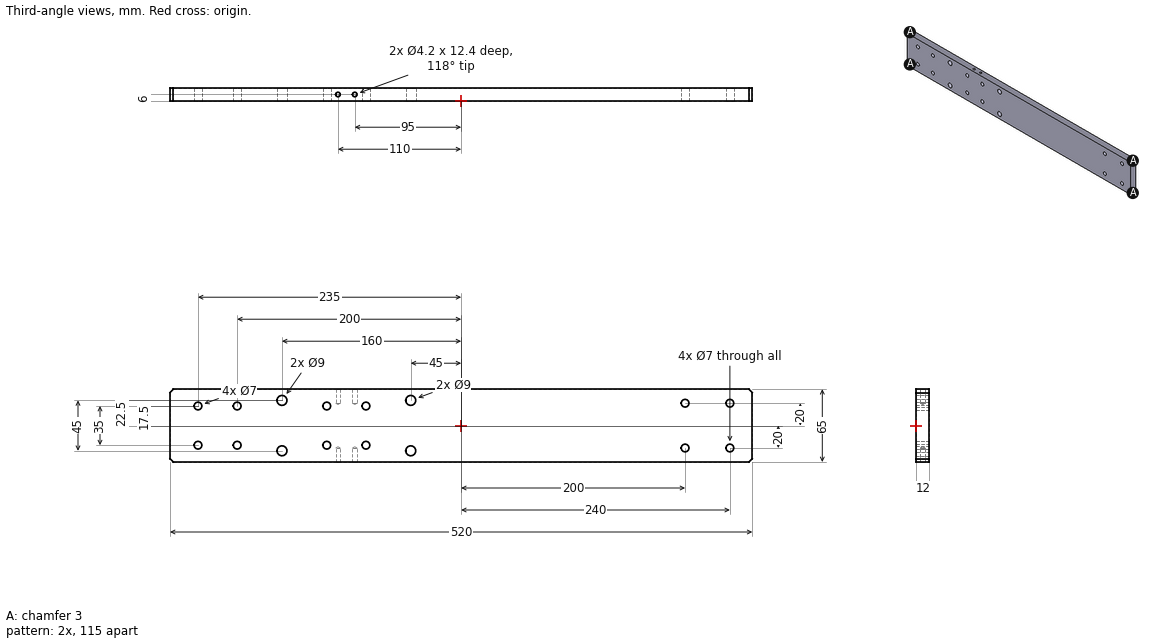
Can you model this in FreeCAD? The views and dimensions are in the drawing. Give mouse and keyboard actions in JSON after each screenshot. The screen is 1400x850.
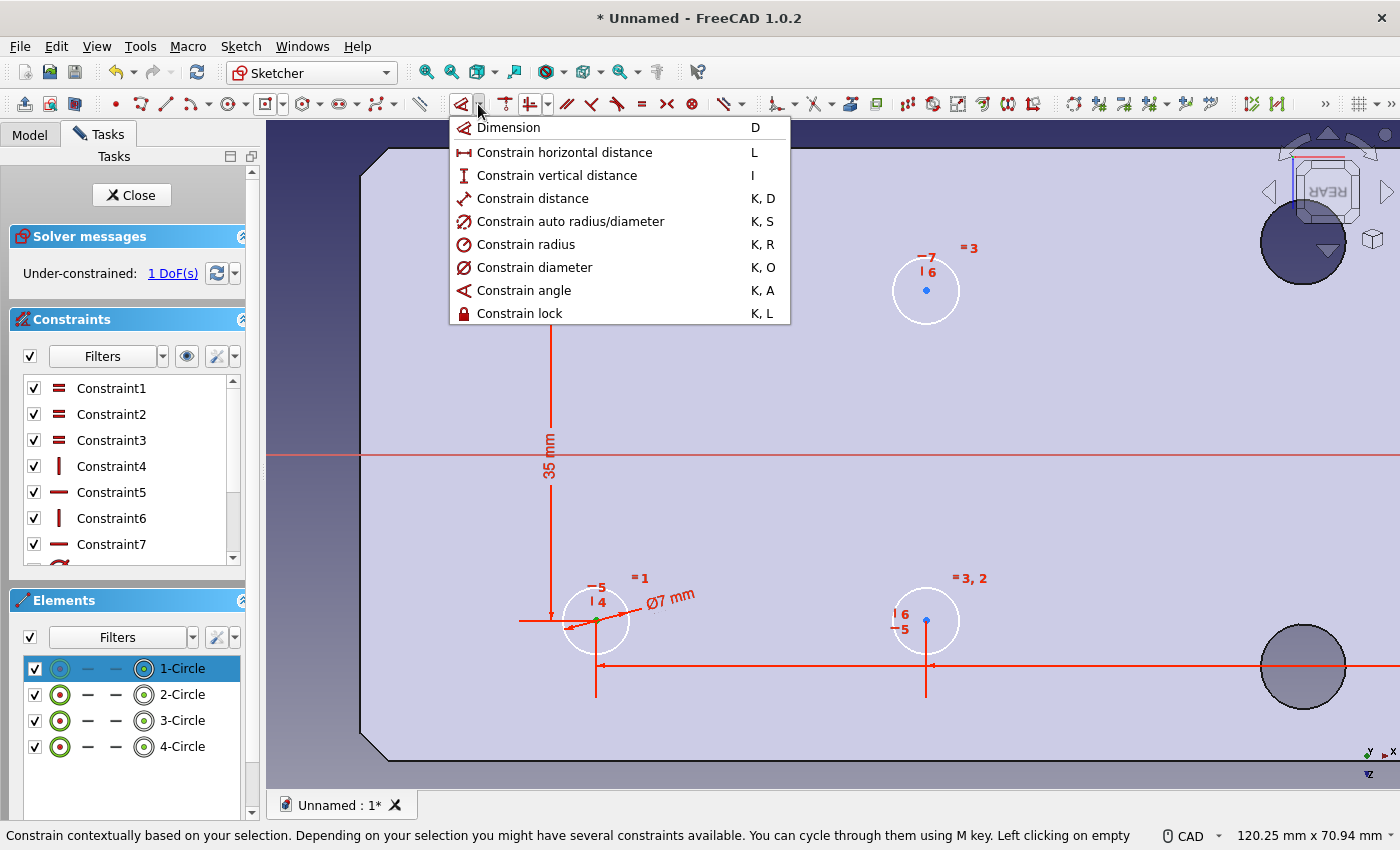
{"action": "left_click", "coordinate": [620, 176]}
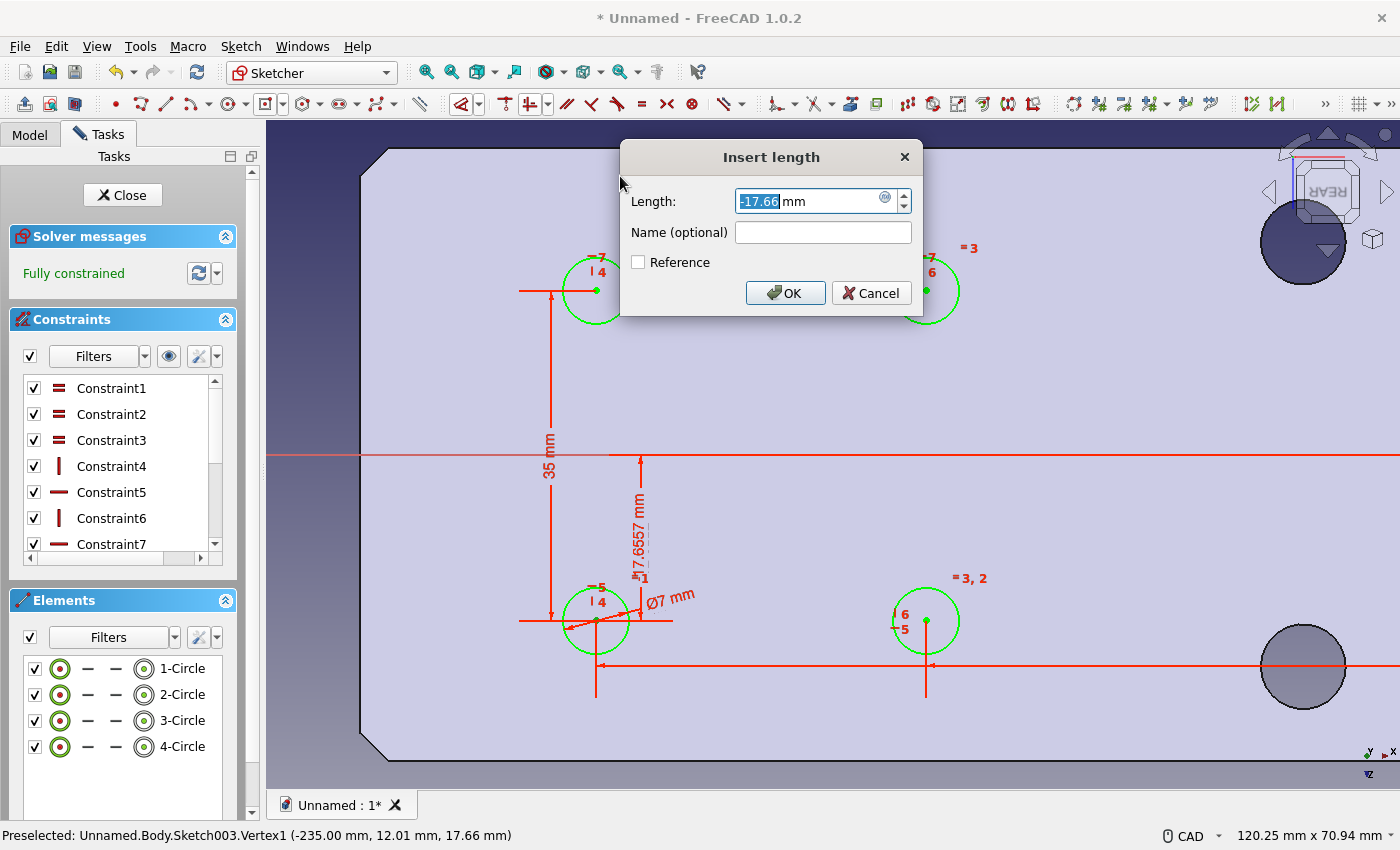
{"action": "type", "text": "-17.5"}
{"action": "key", "text": "Return"}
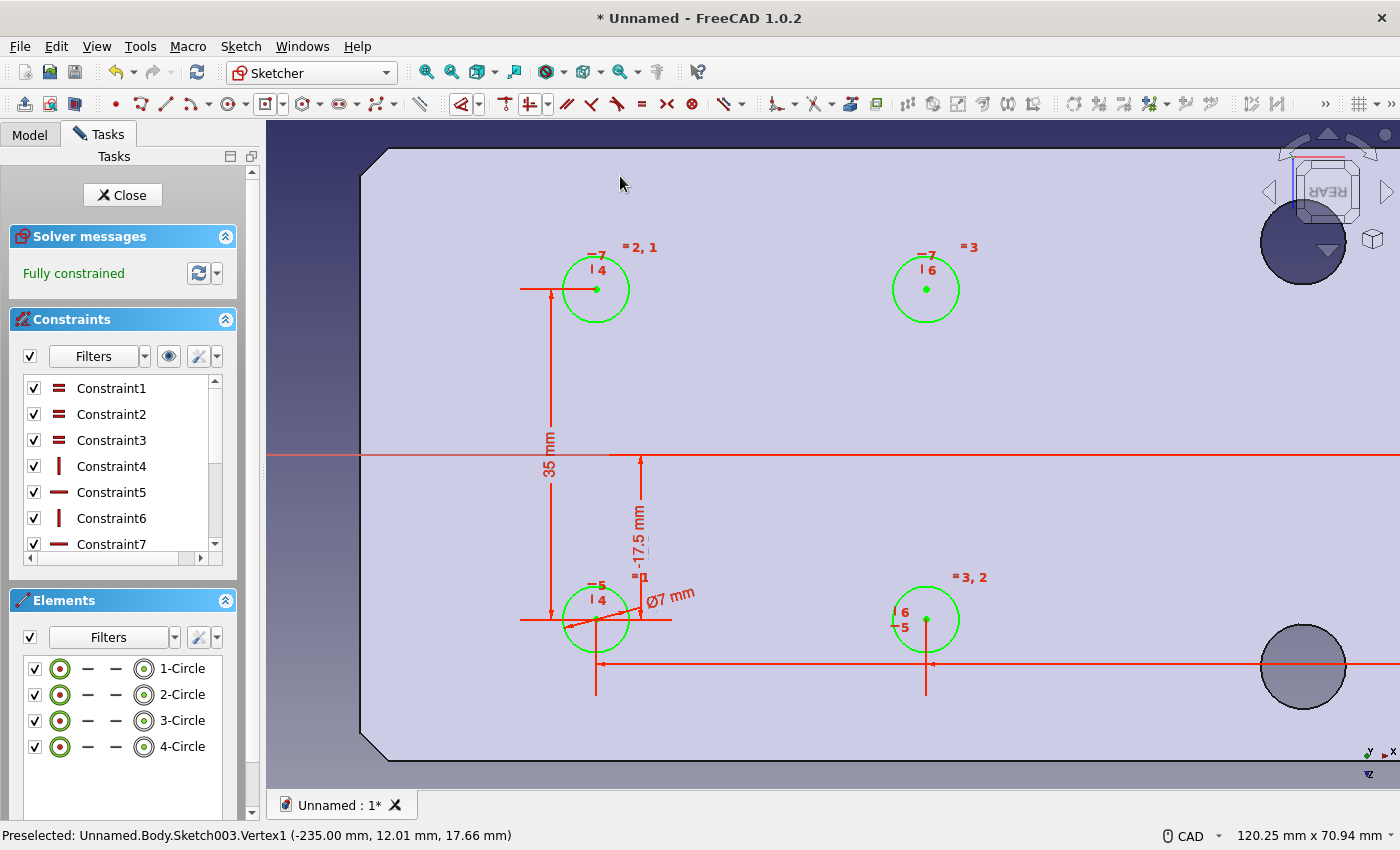
{"action": "left_click", "coordinate": [123, 195]}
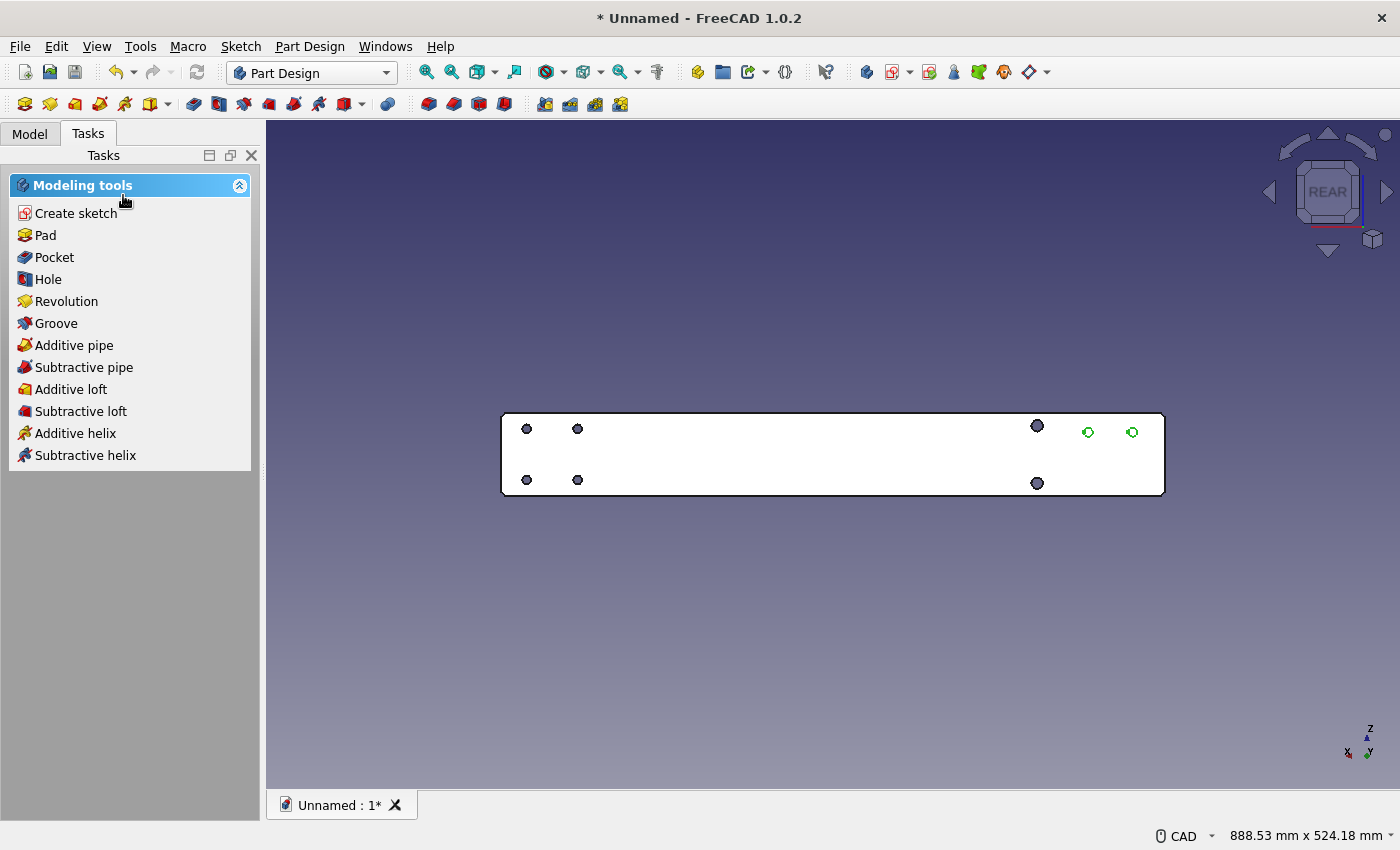
{"action": "left_click", "coordinate": [194, 104]}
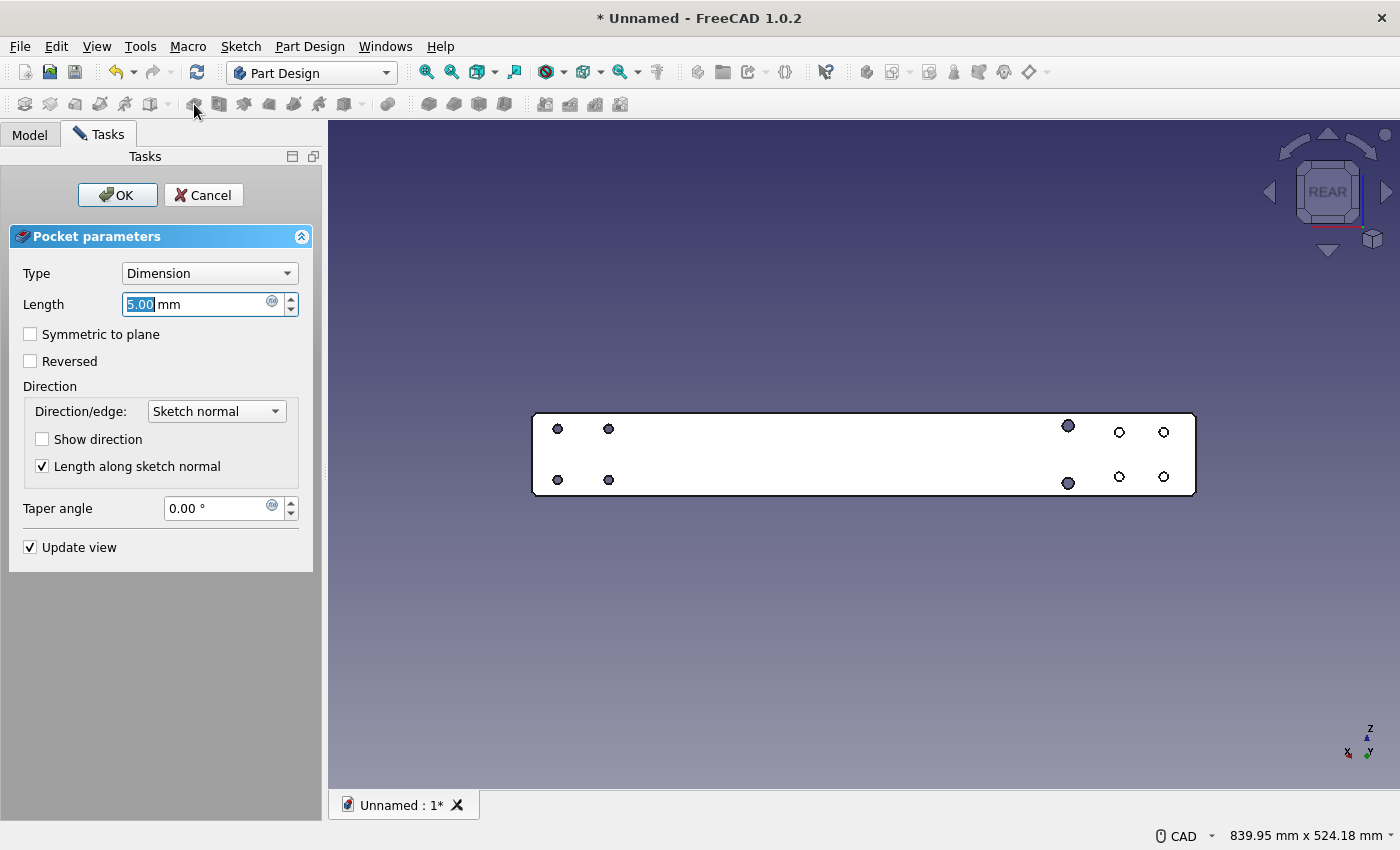
{"action": "left_click", "coordinate": [210, 274]}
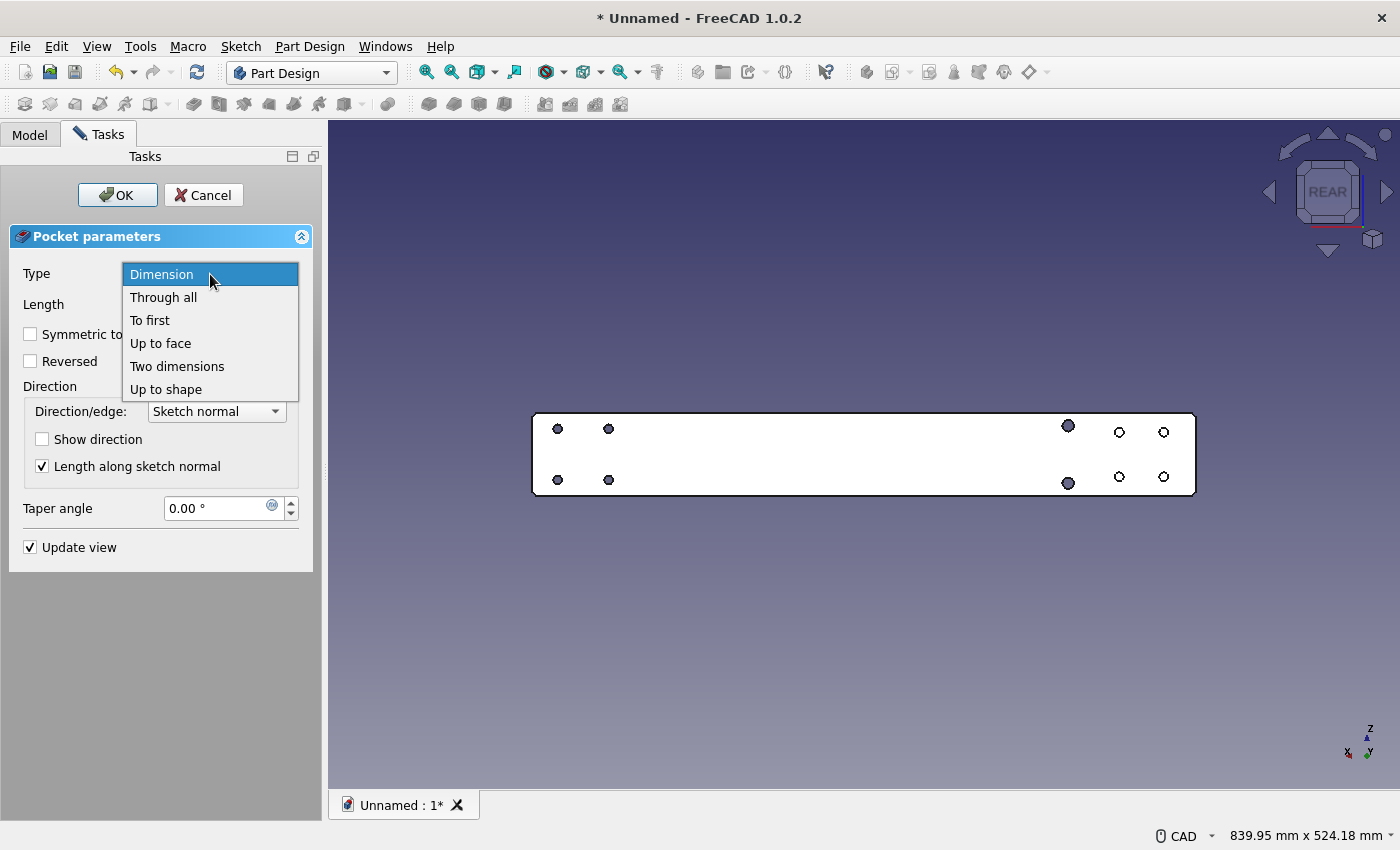
{"action": "left_click", "coordinate": [208, 298]}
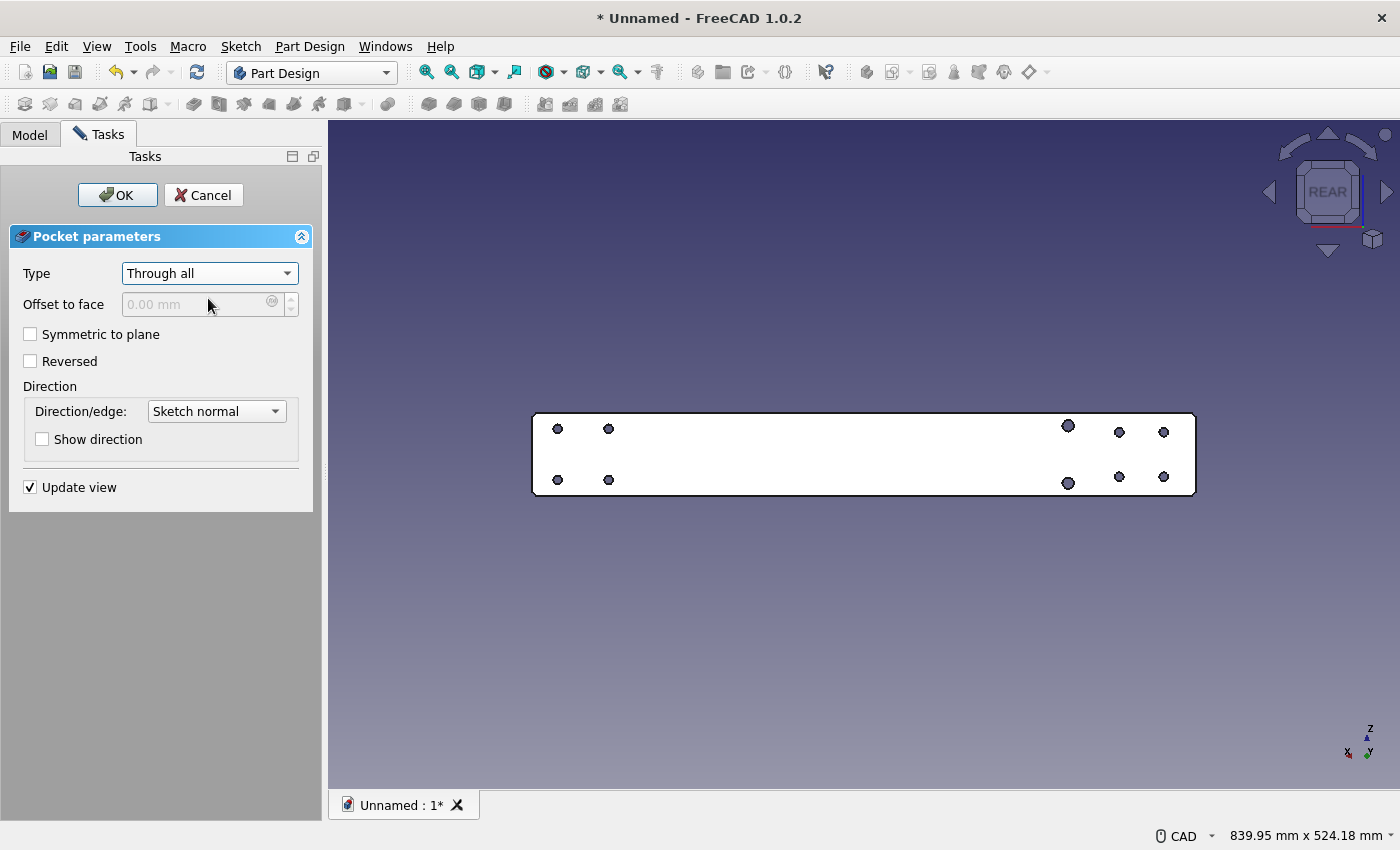
{"action": "left_click", "coordinate": [118, 195]}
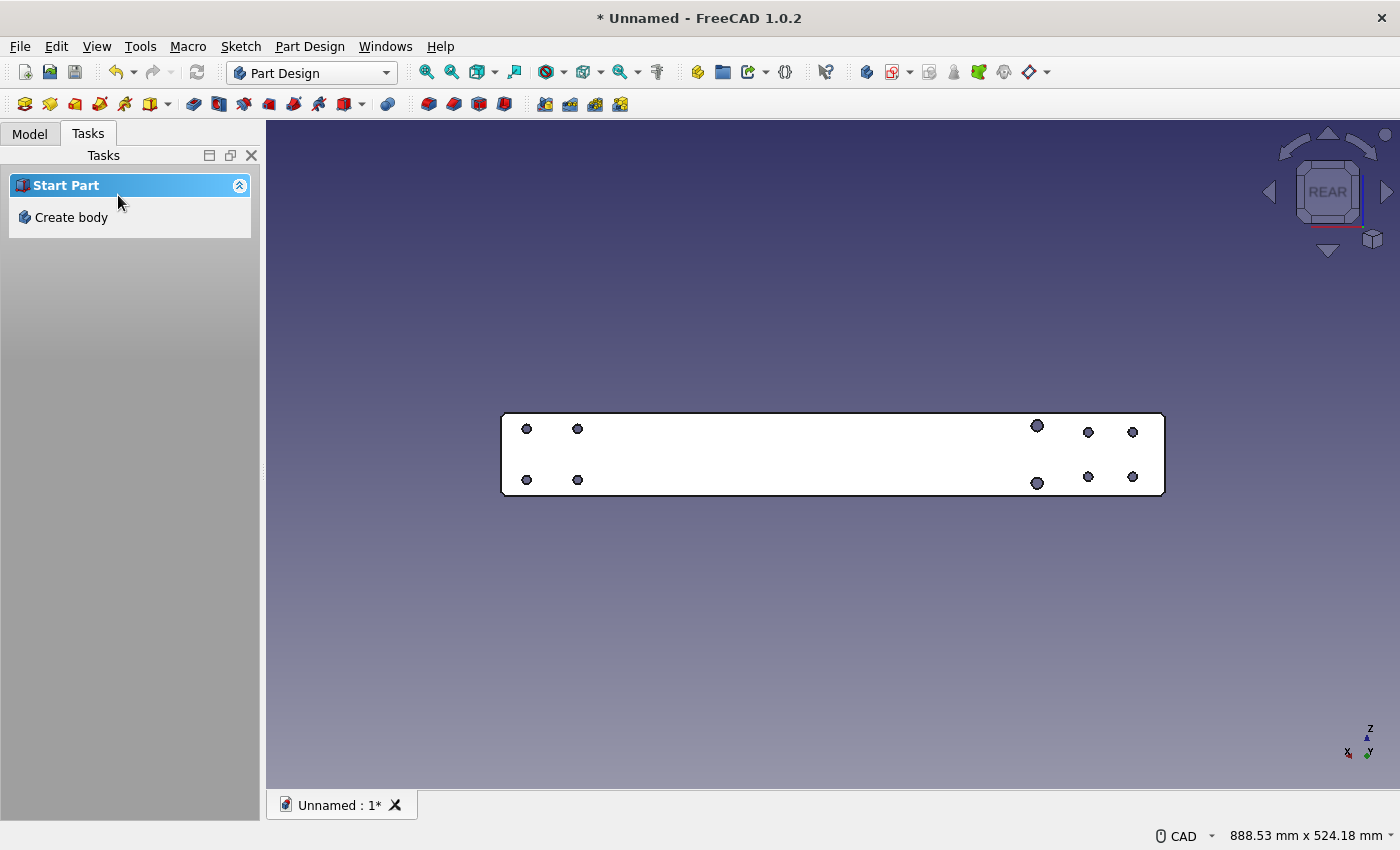
{"action": "left_click", "coordinate": [30, 134]}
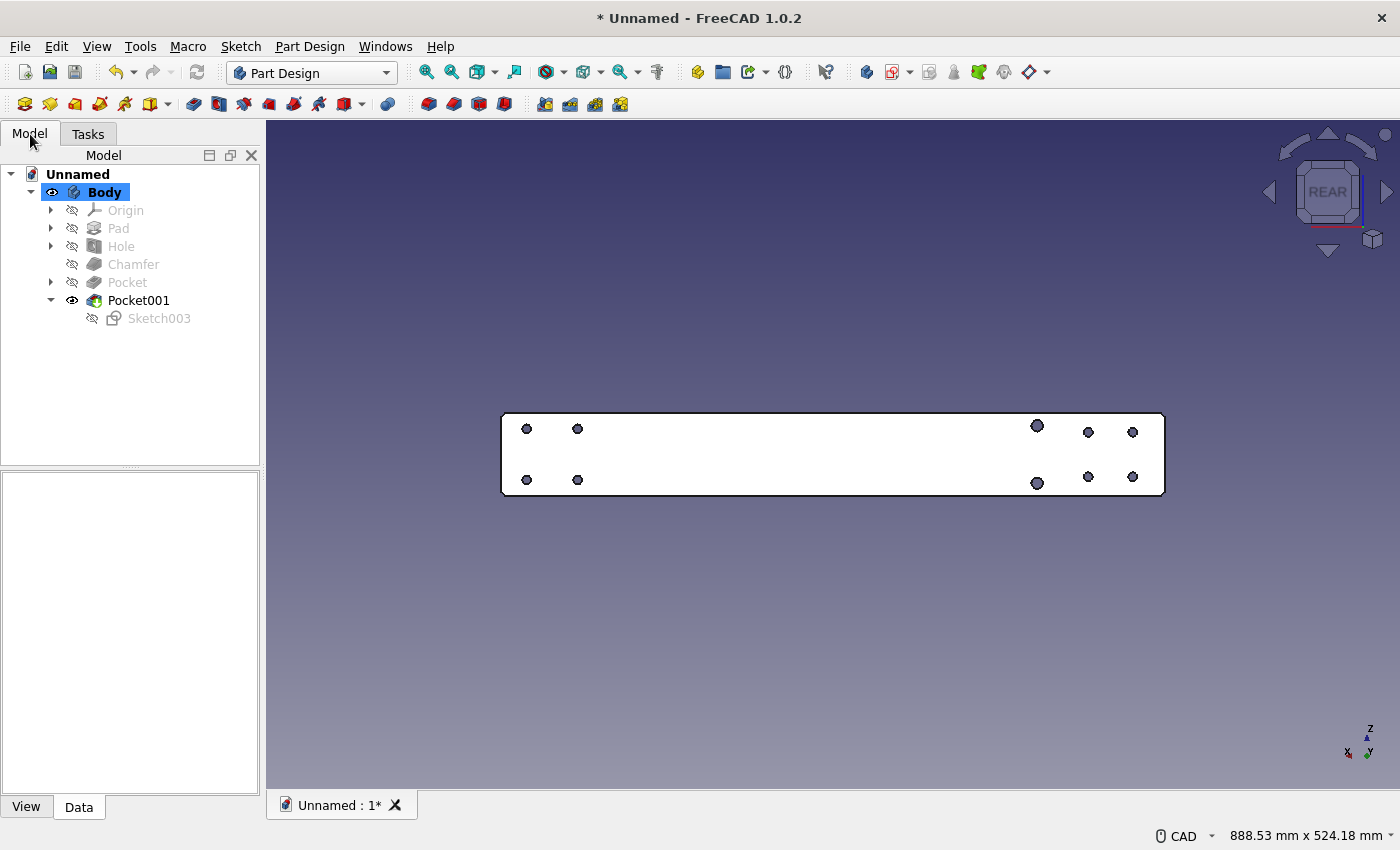
{"action": "left_click", "coordinate": [117, 300]}